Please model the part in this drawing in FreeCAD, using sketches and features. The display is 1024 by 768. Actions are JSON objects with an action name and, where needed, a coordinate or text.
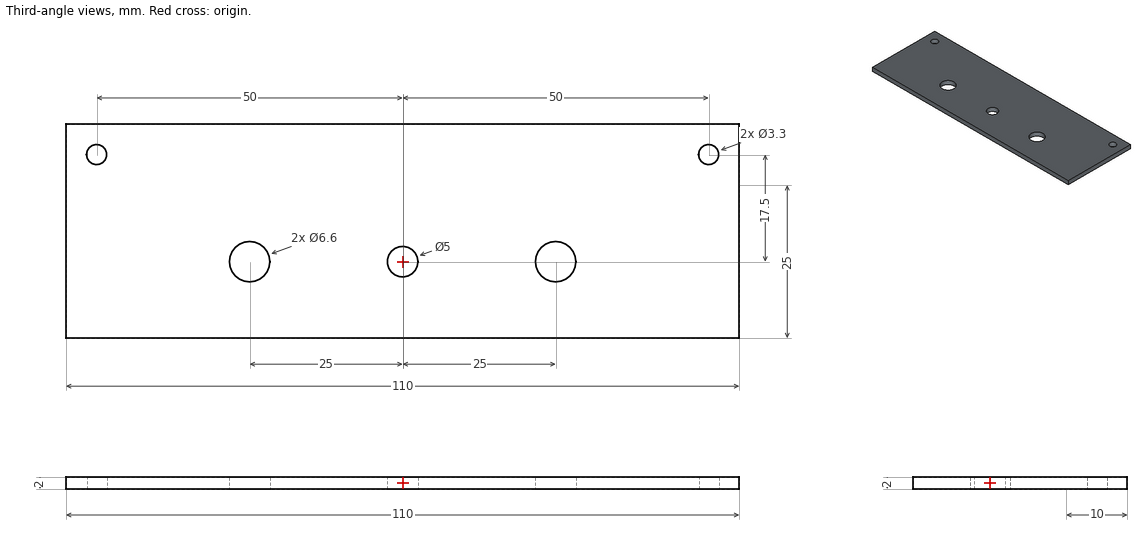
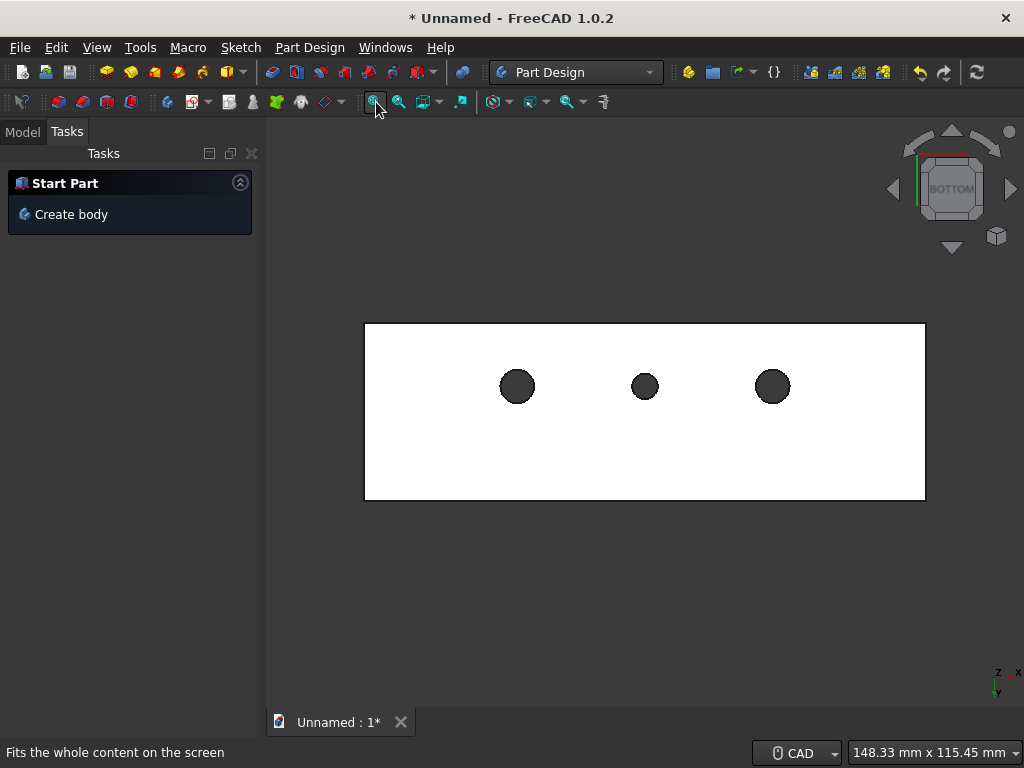
{"action": "left_click", "coordinate": [565, 437]}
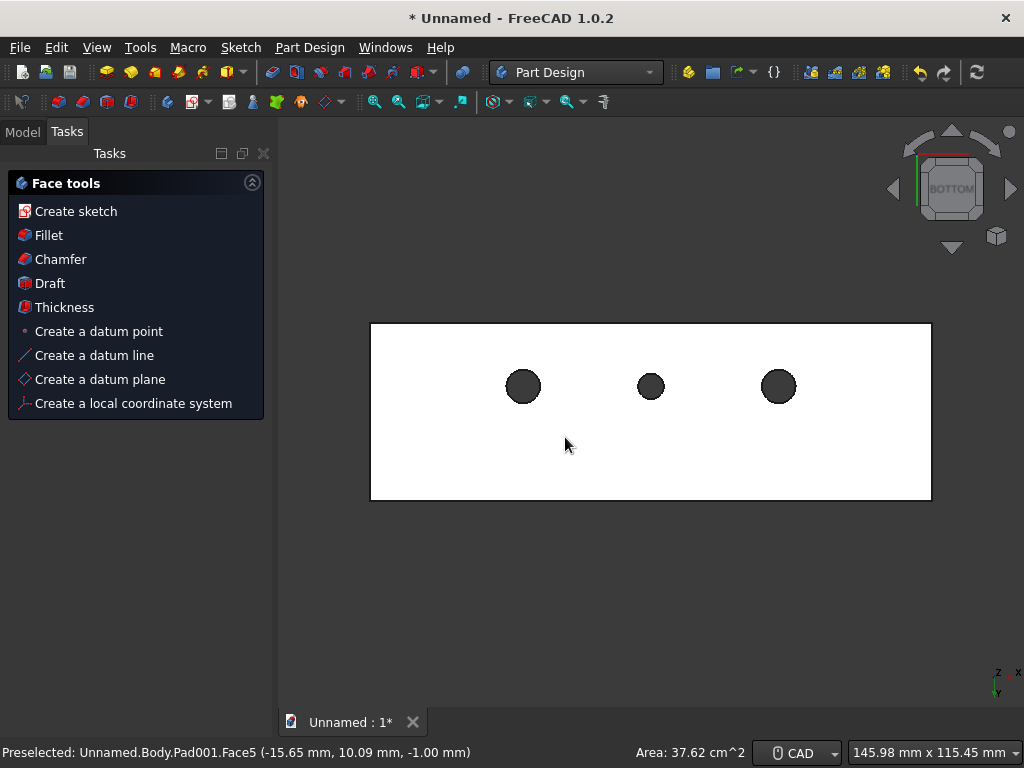
{"action": "left_click", "coordinate": [192, 102]}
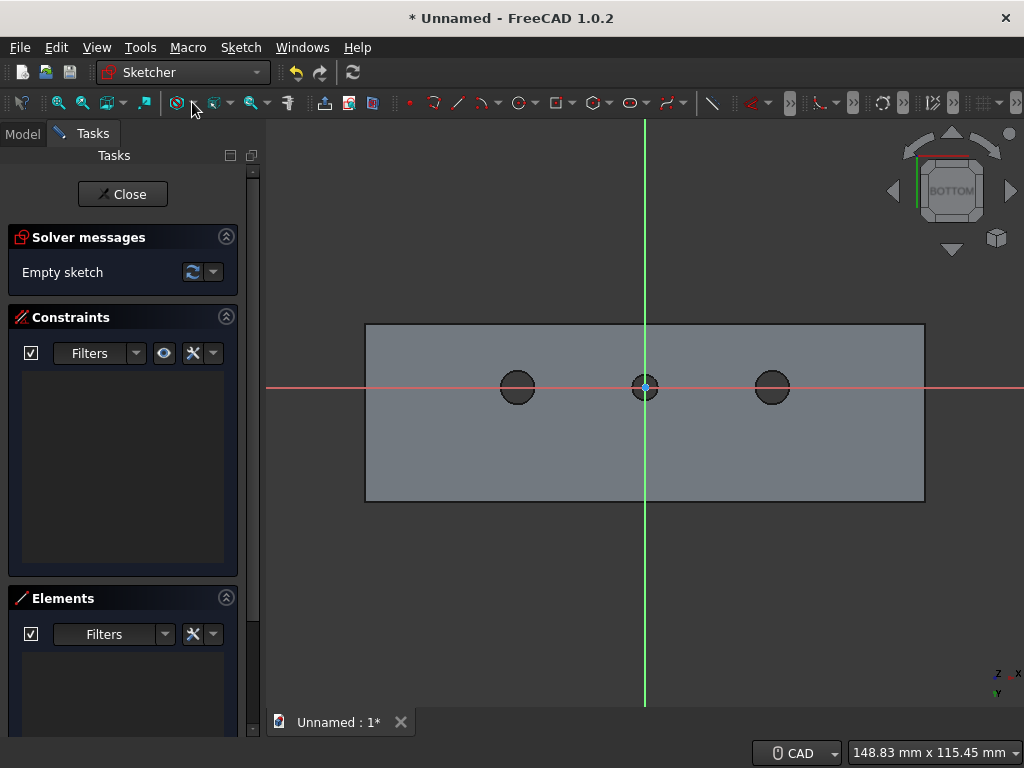
{"action": "scroll", "coordinate": [294, 308], "scroll_direction": "down", "scroll_amount": 1}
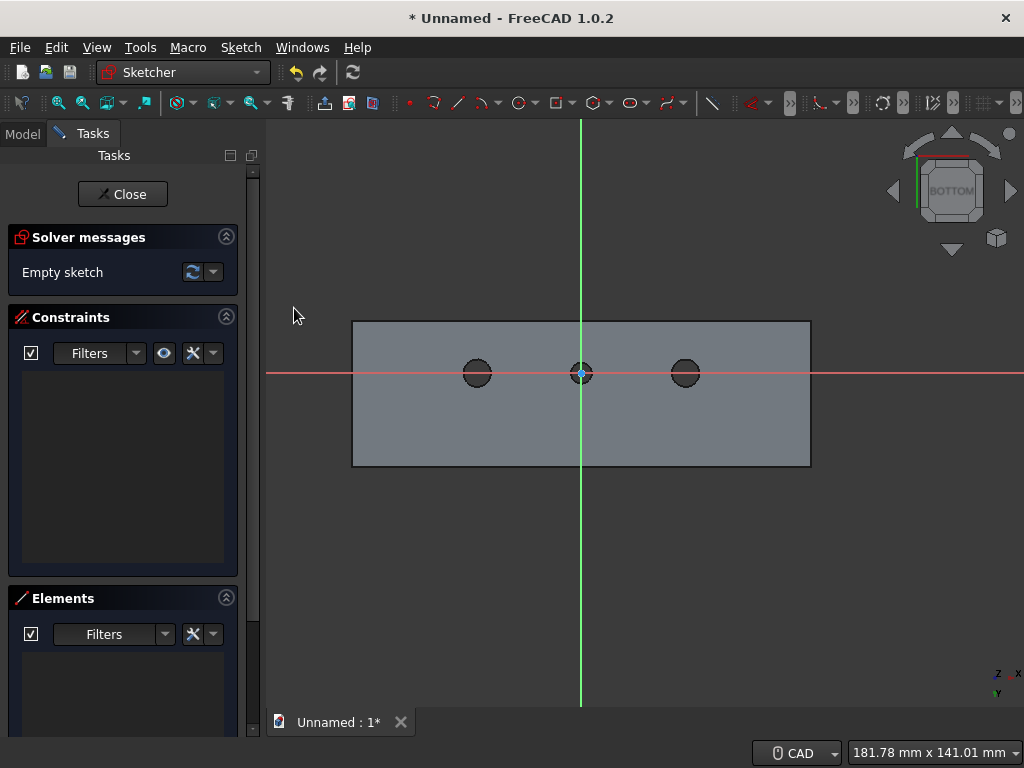
{"action": "key", "text": "g c"}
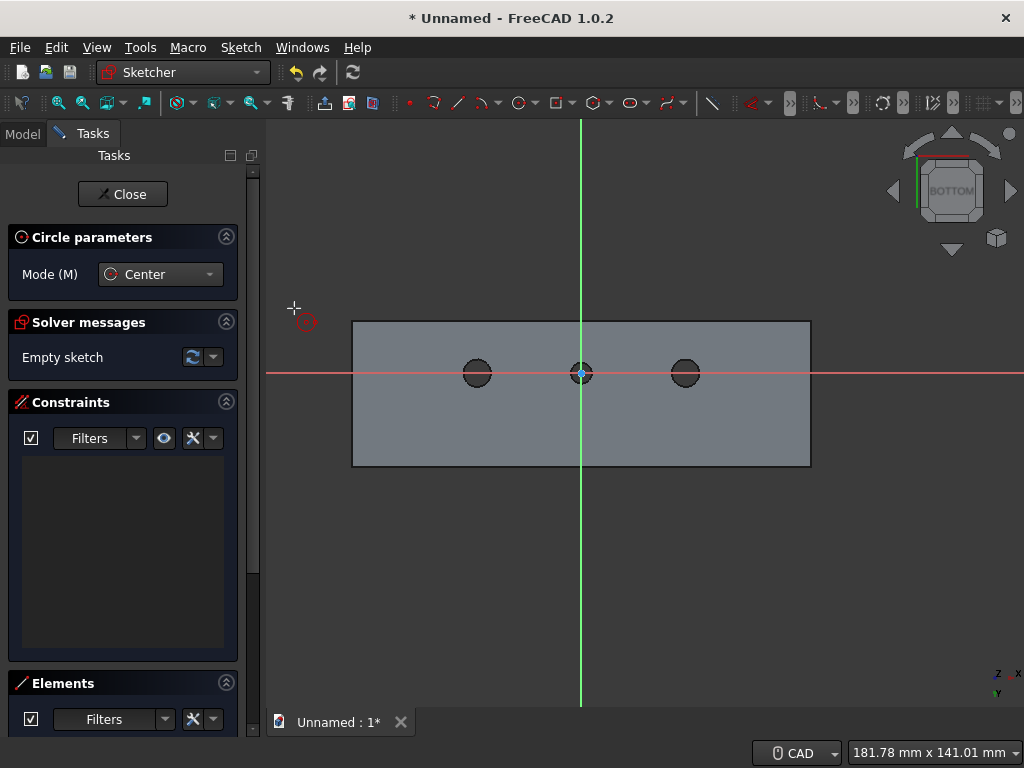
{"action": "scroll", "coordinate": [790, 446], "scroll_direction": "up", "scroll_amount": 6}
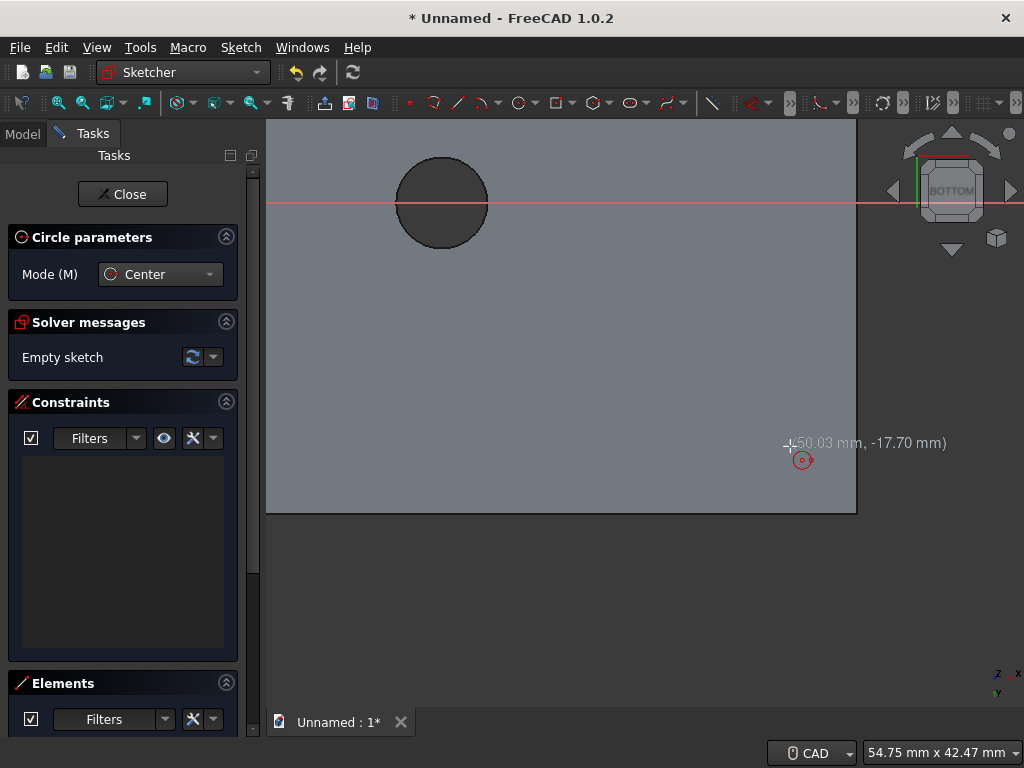
{"action": "left_click", "coordinate": [788, 445]}
{"action": "mouse_move", "coordinate": [804, 429]}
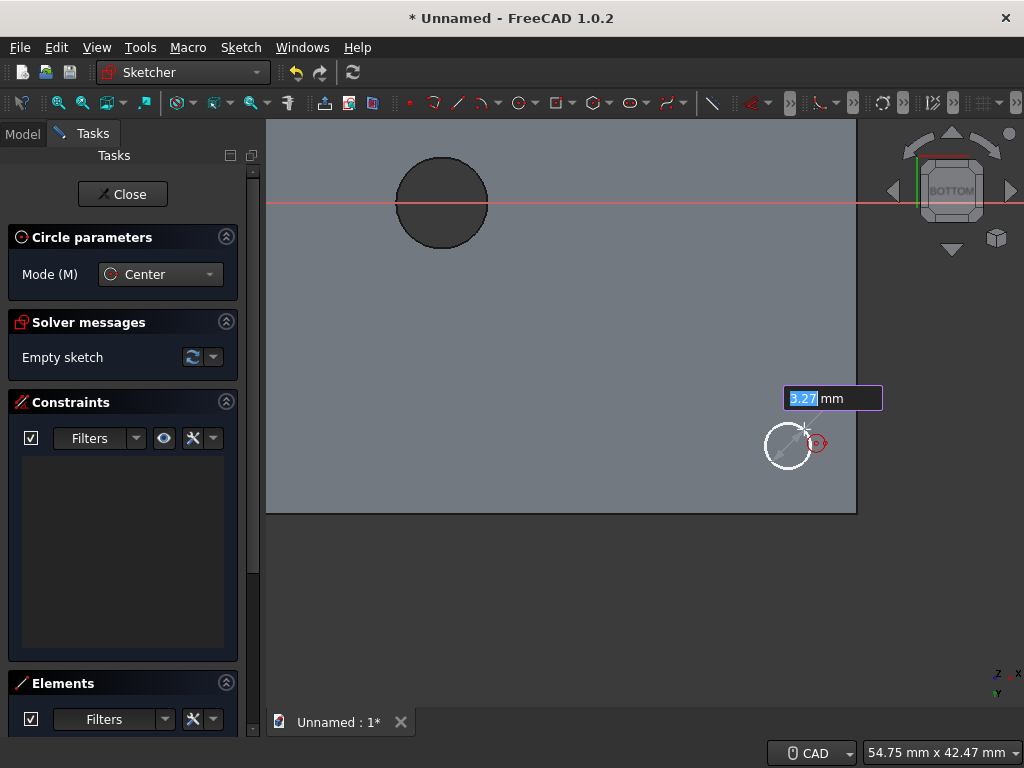
{"action": "type", "text": "3.3"}
{"action": "key", "text": "Return"}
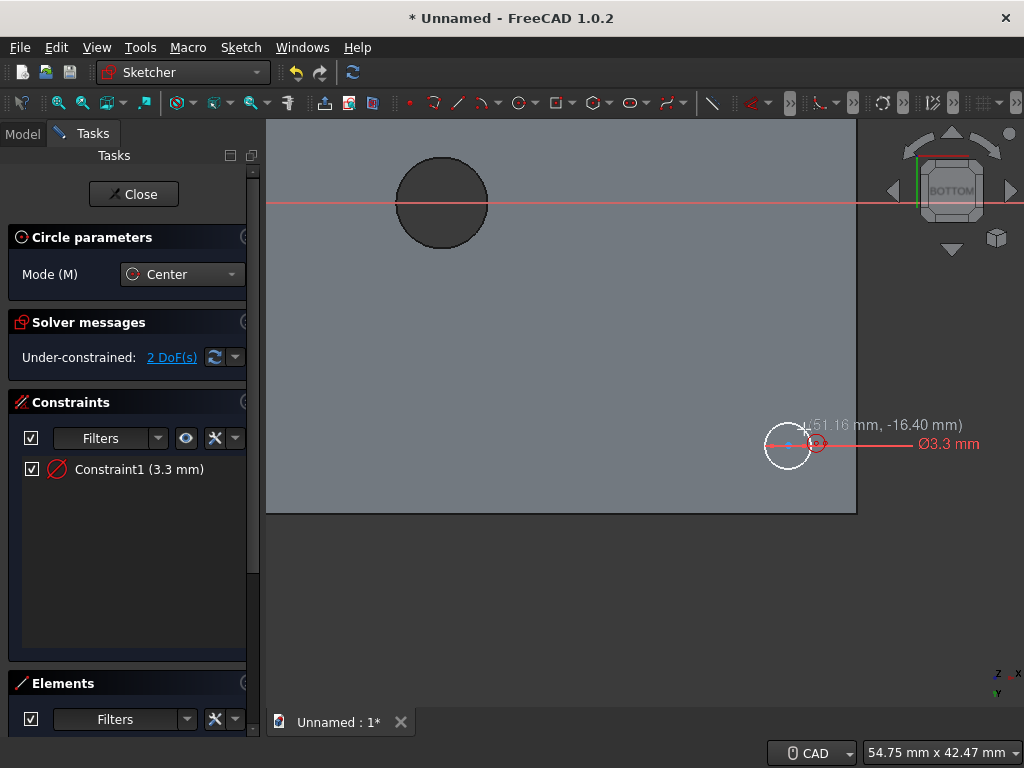
{"action": "scroll", "coordinate": [784, 446], "scroll_direction": "down", "scroll_amount": 6}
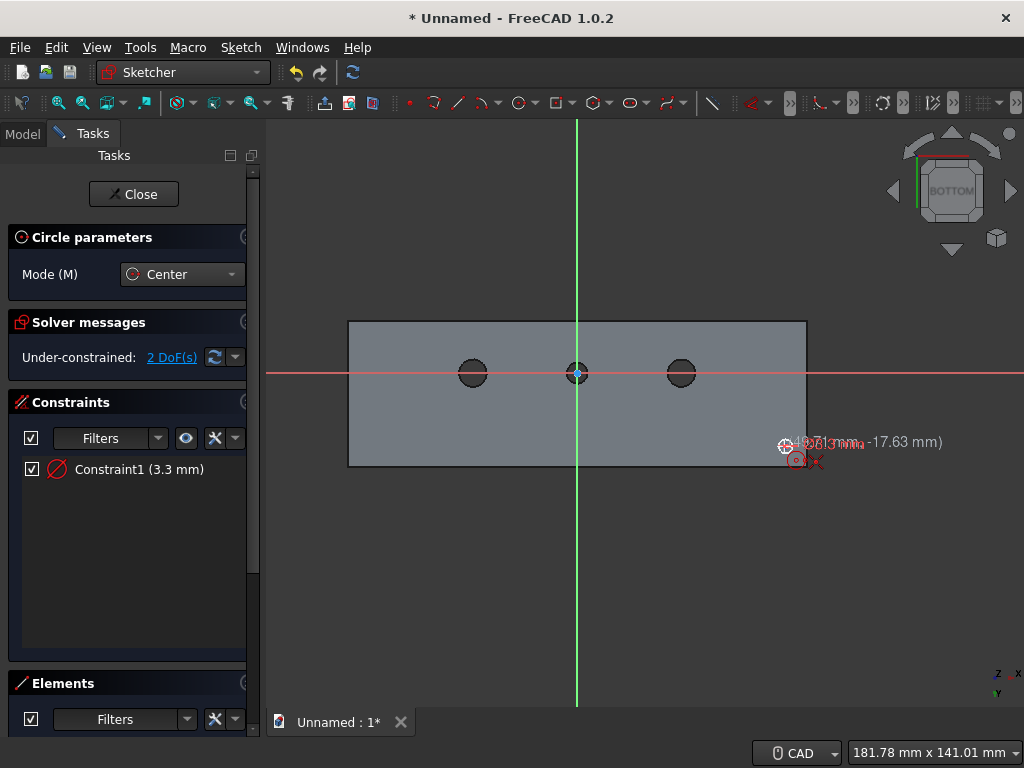
{"action": "scroll", "coordinate": [369, 446], "scroll_direction": "up", "scroll_amount": 6}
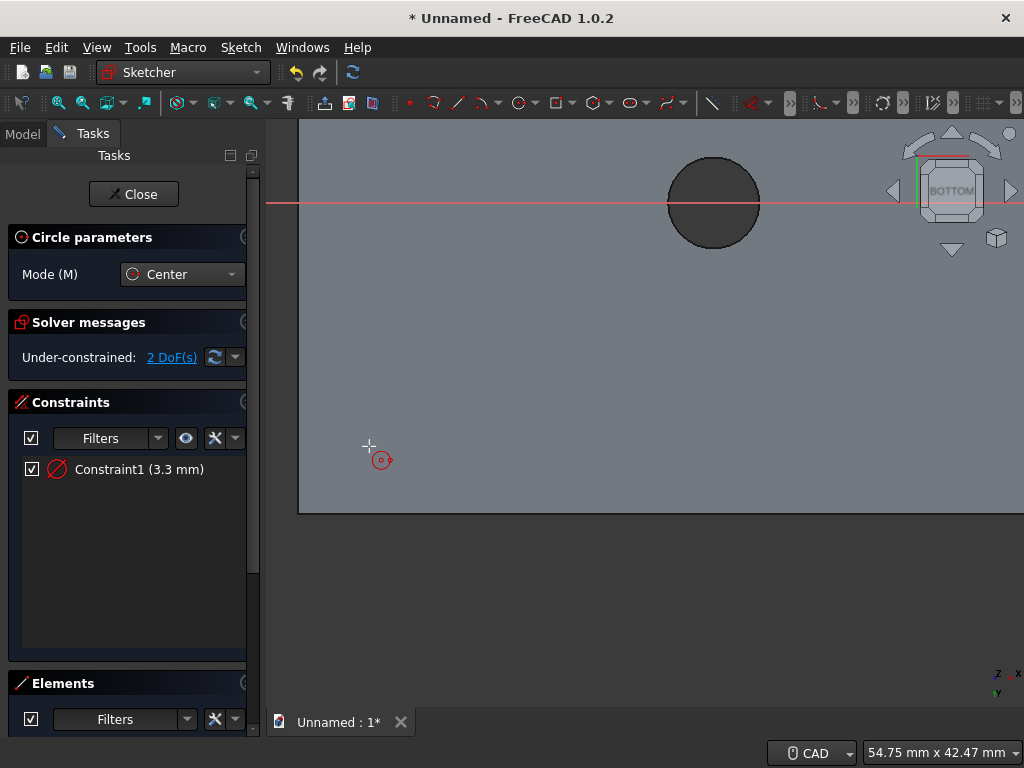
{"action": "left_click", "coordinate": [368, 445]}
{"action": "mouse_move", "coordinate": [384, 429]}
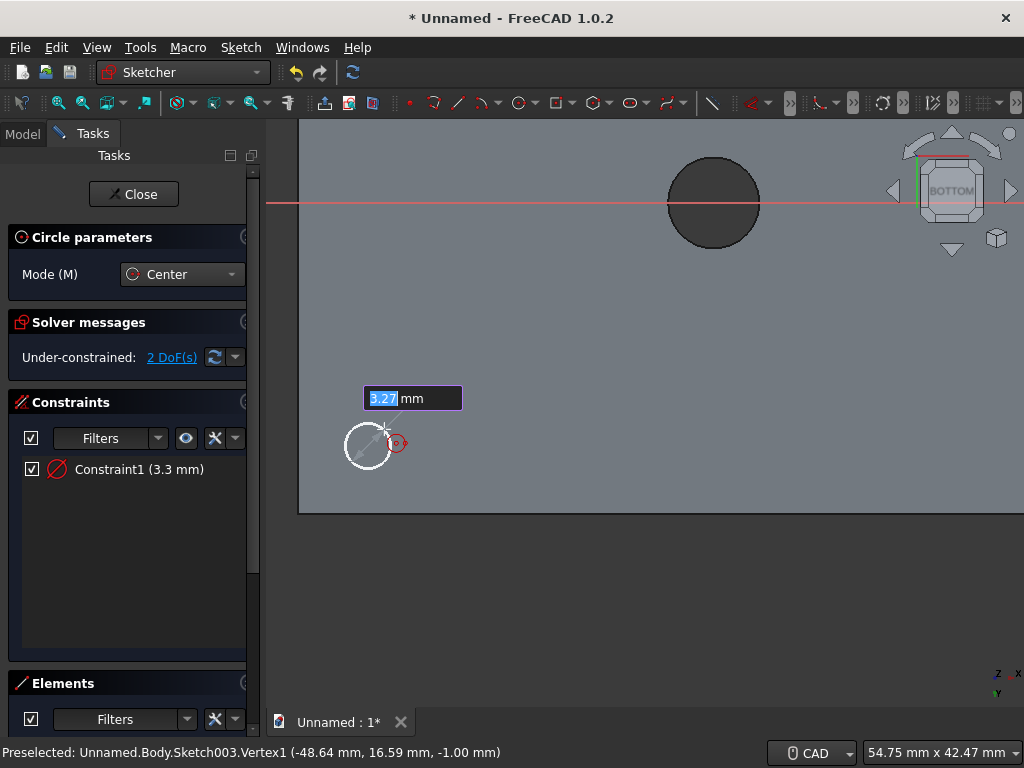
{"action": "type", "text": "3.3"}
{"action": "key", "text": "Return"}
{"action": "key", "text": "Escape"}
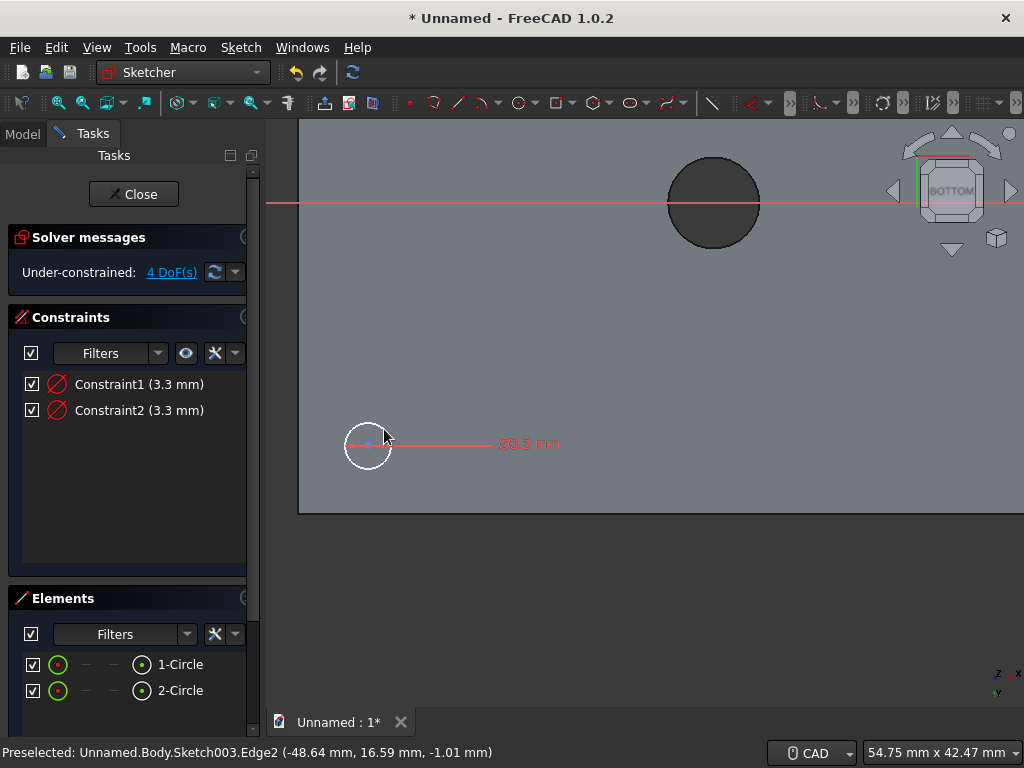
{"action": "scroll", "coordinate": [368, 446], "scroll_direction": "down", "scroll_amount": 6}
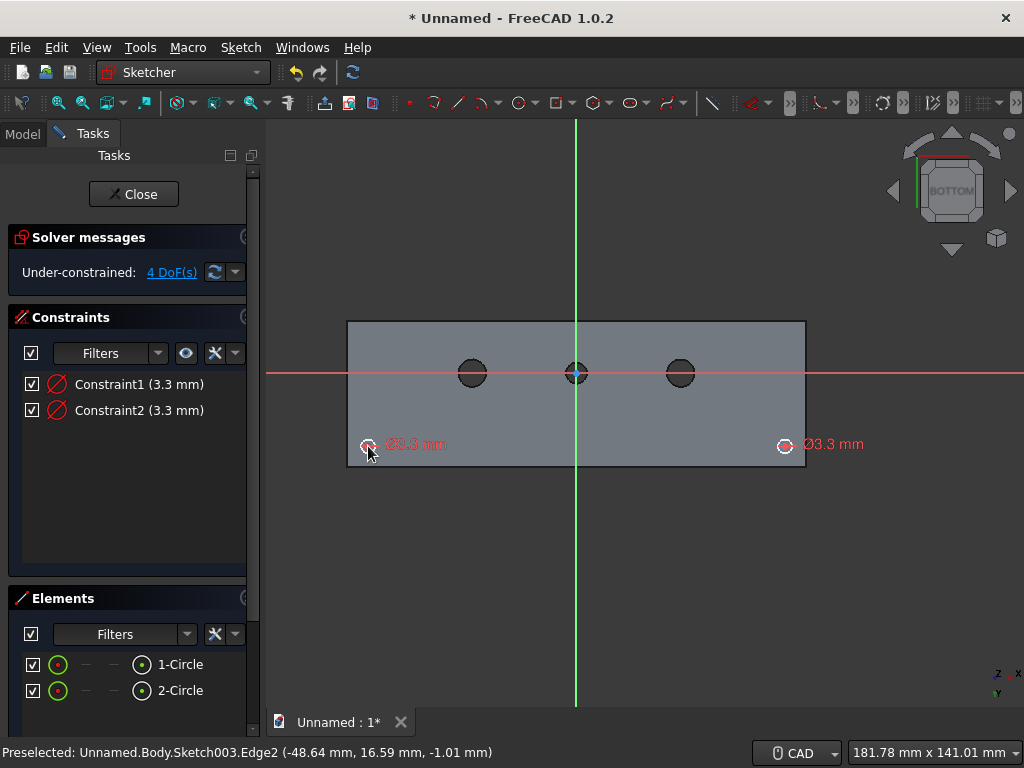
{"action": "left_click", "coordinate": [785, 446]}